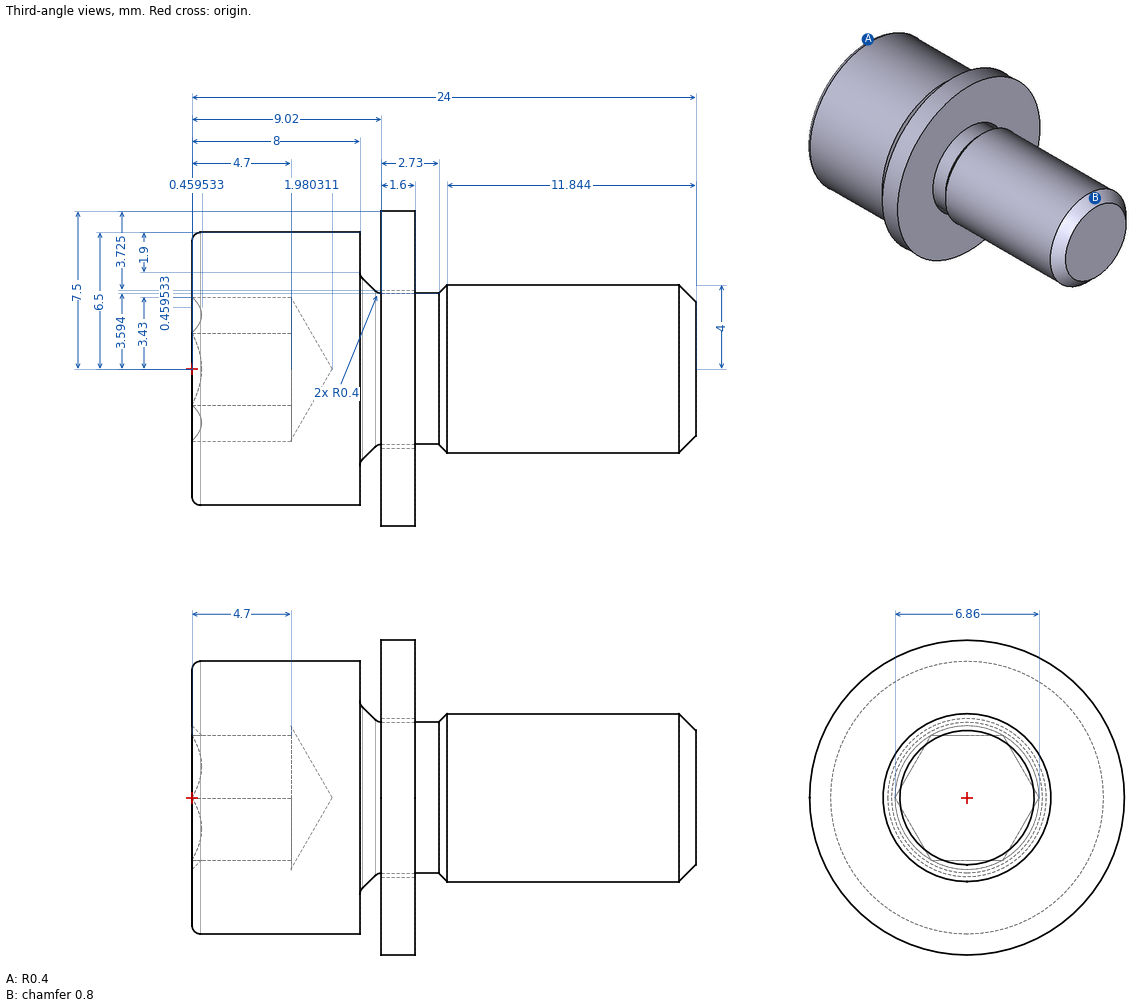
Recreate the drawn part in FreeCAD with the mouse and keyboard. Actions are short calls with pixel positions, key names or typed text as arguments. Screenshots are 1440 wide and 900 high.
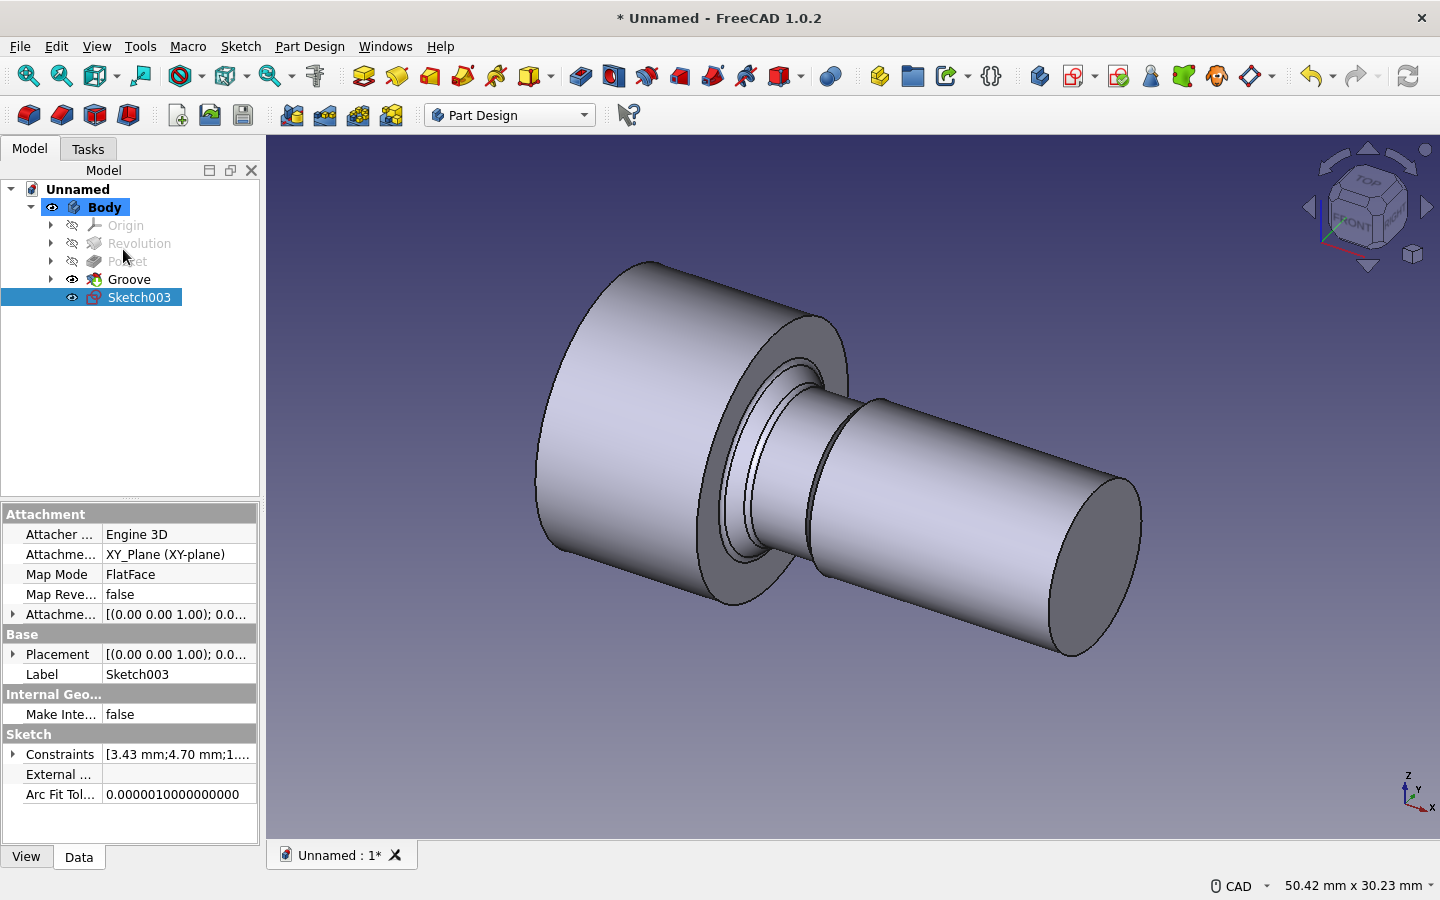
click(647, 76)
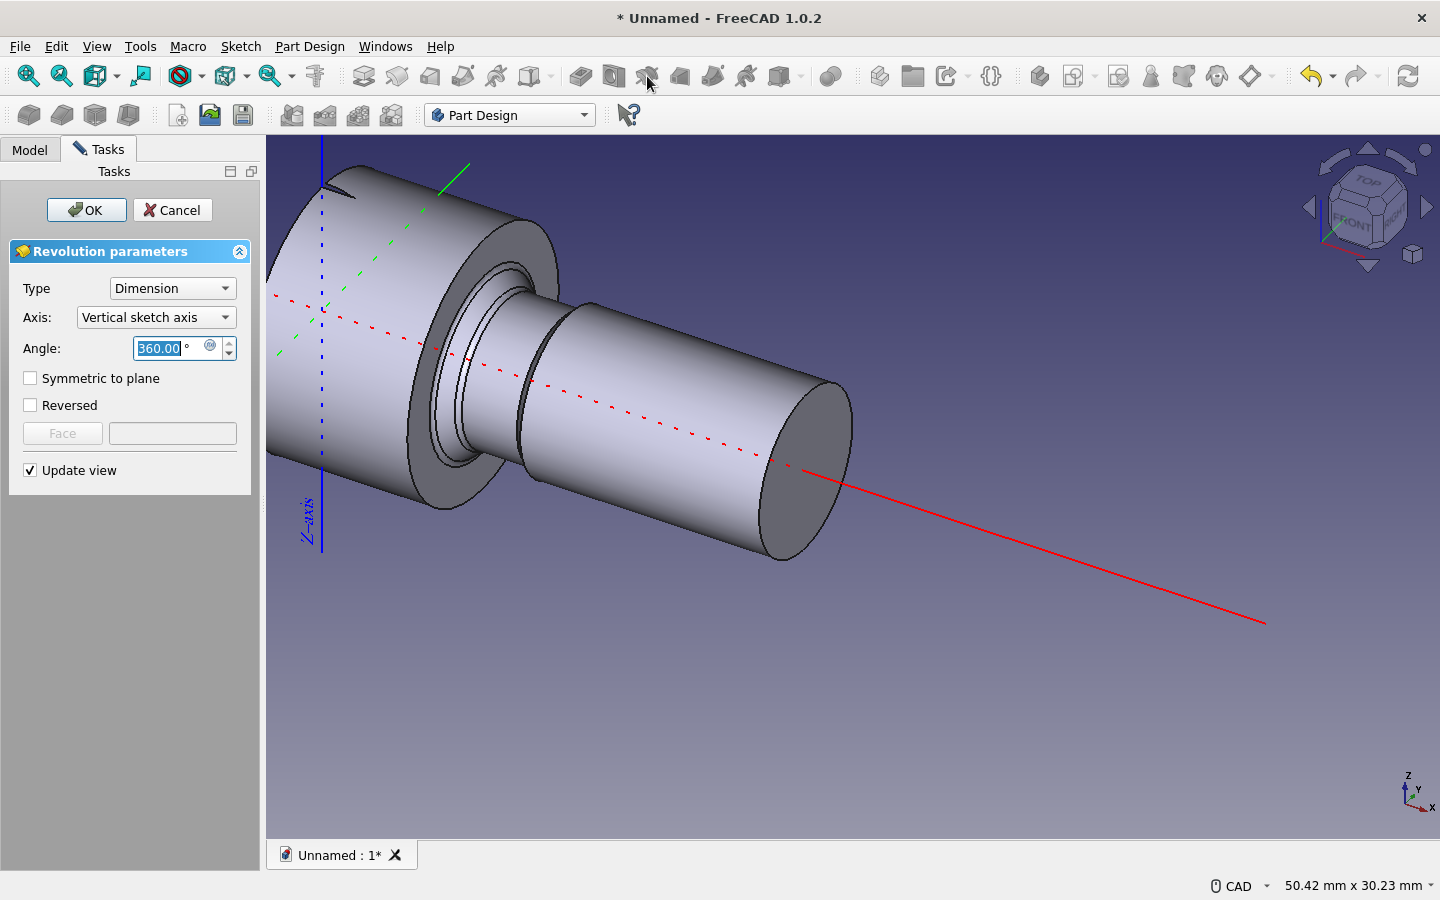
click(157, 318)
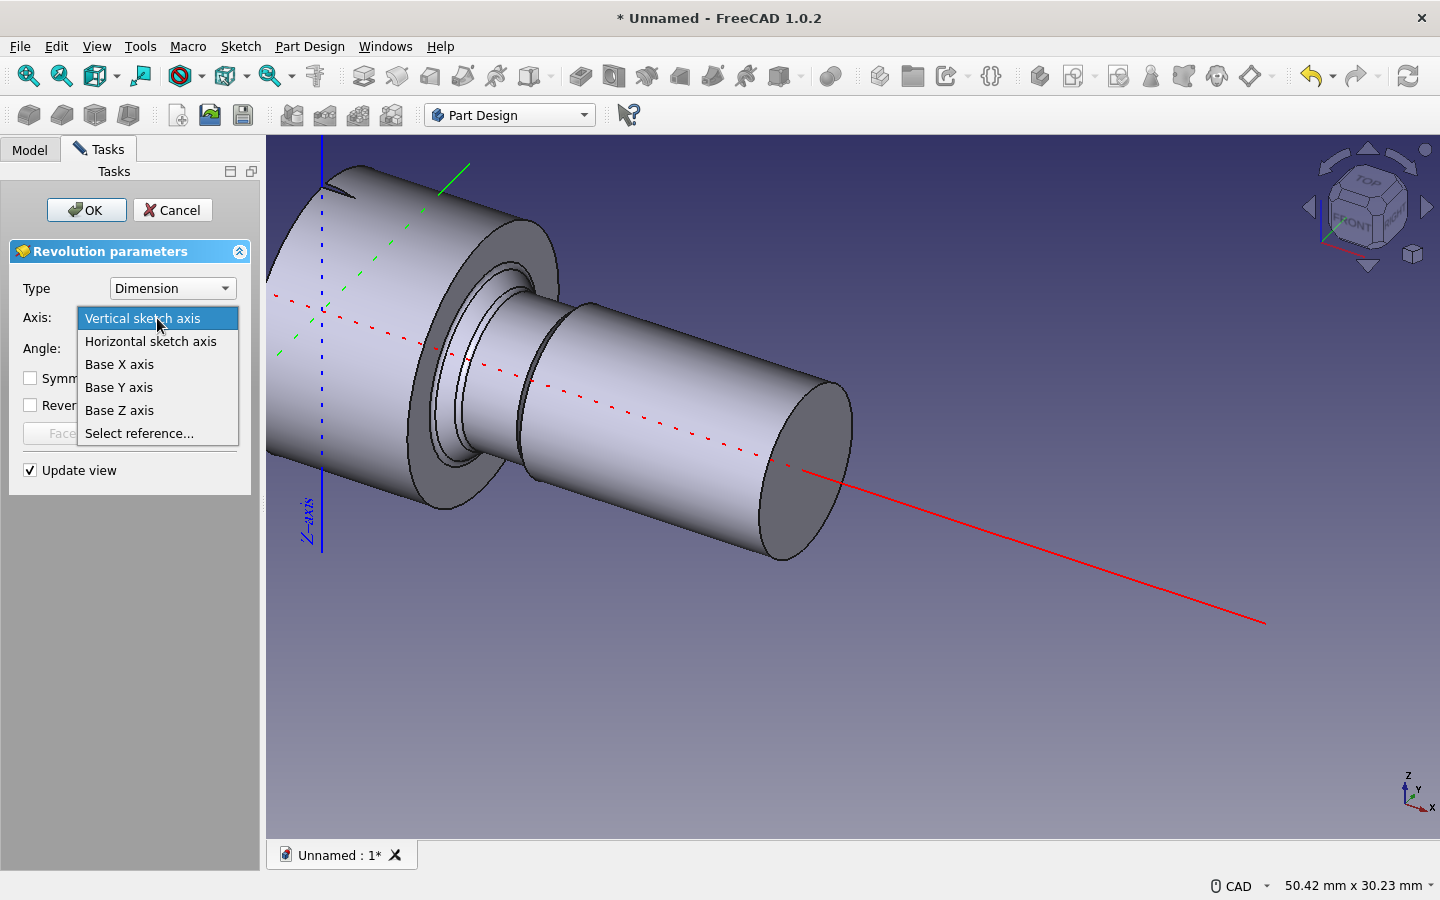
click(156, 342)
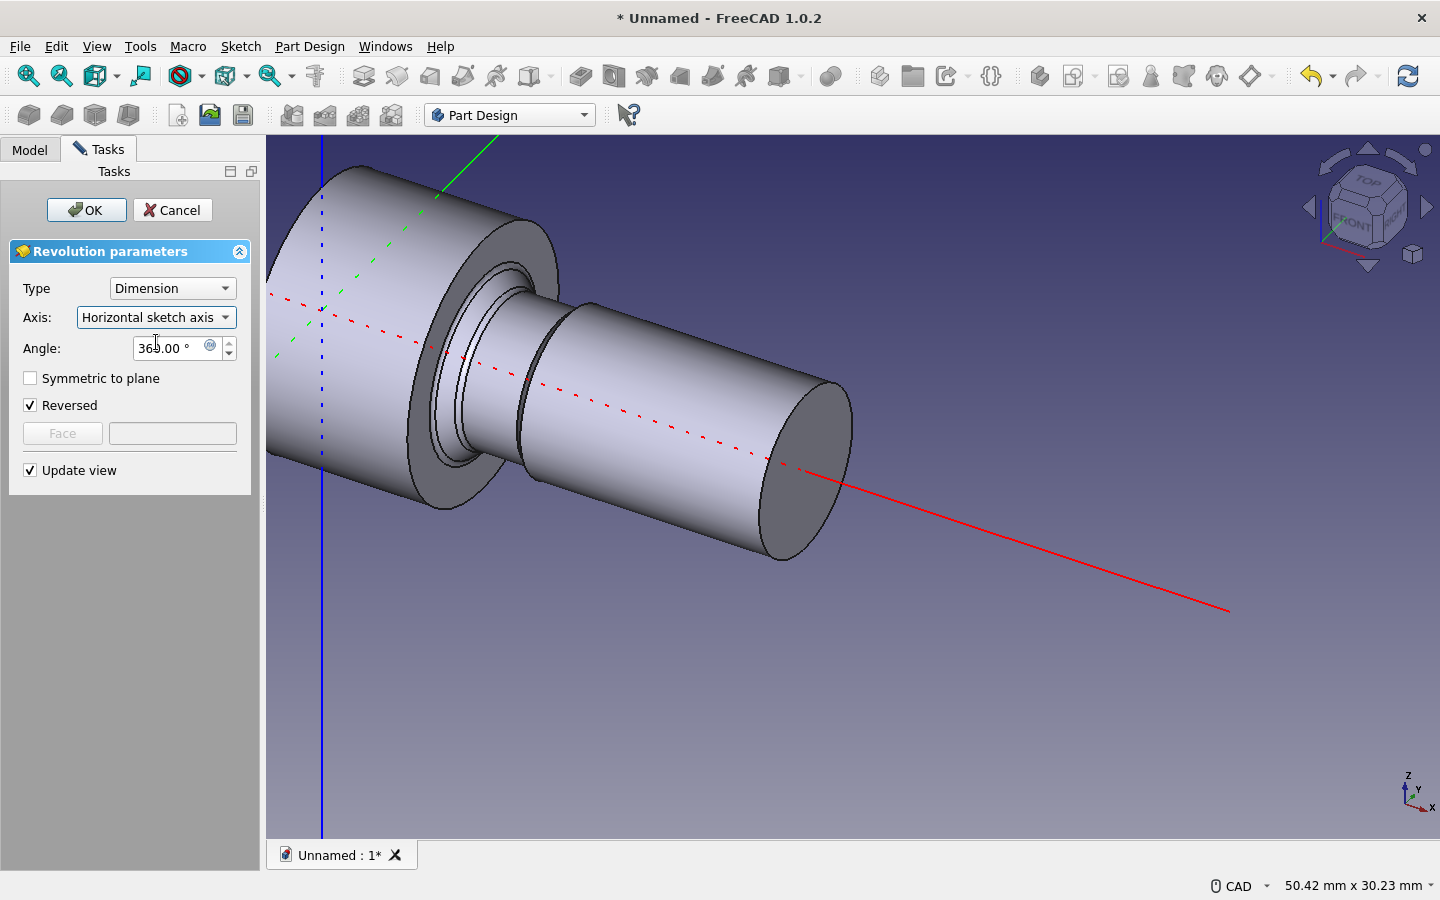
click(87, 210)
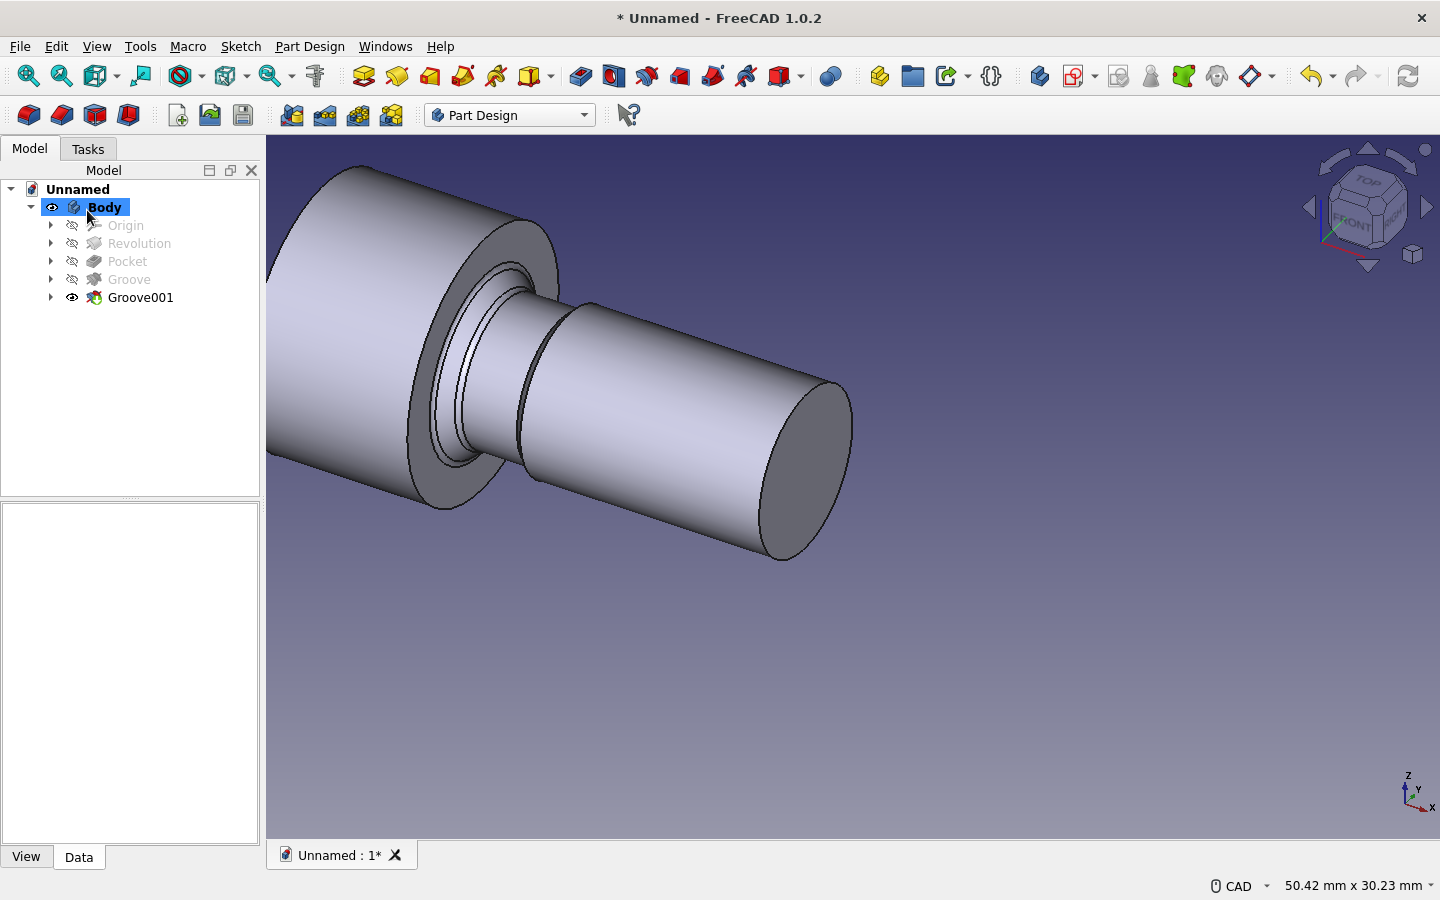
click(29, 76)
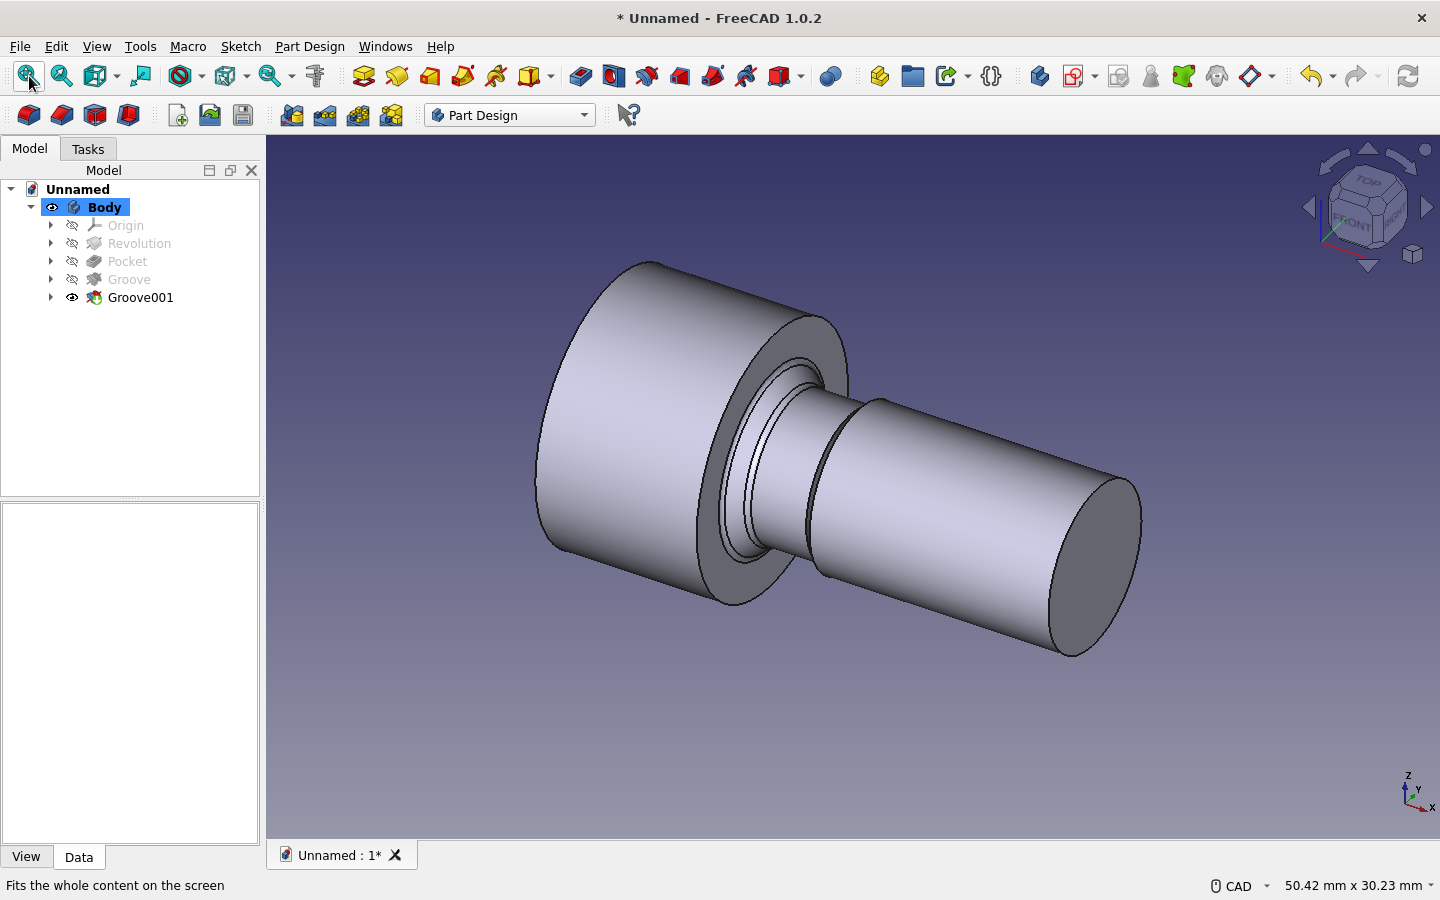
key(0)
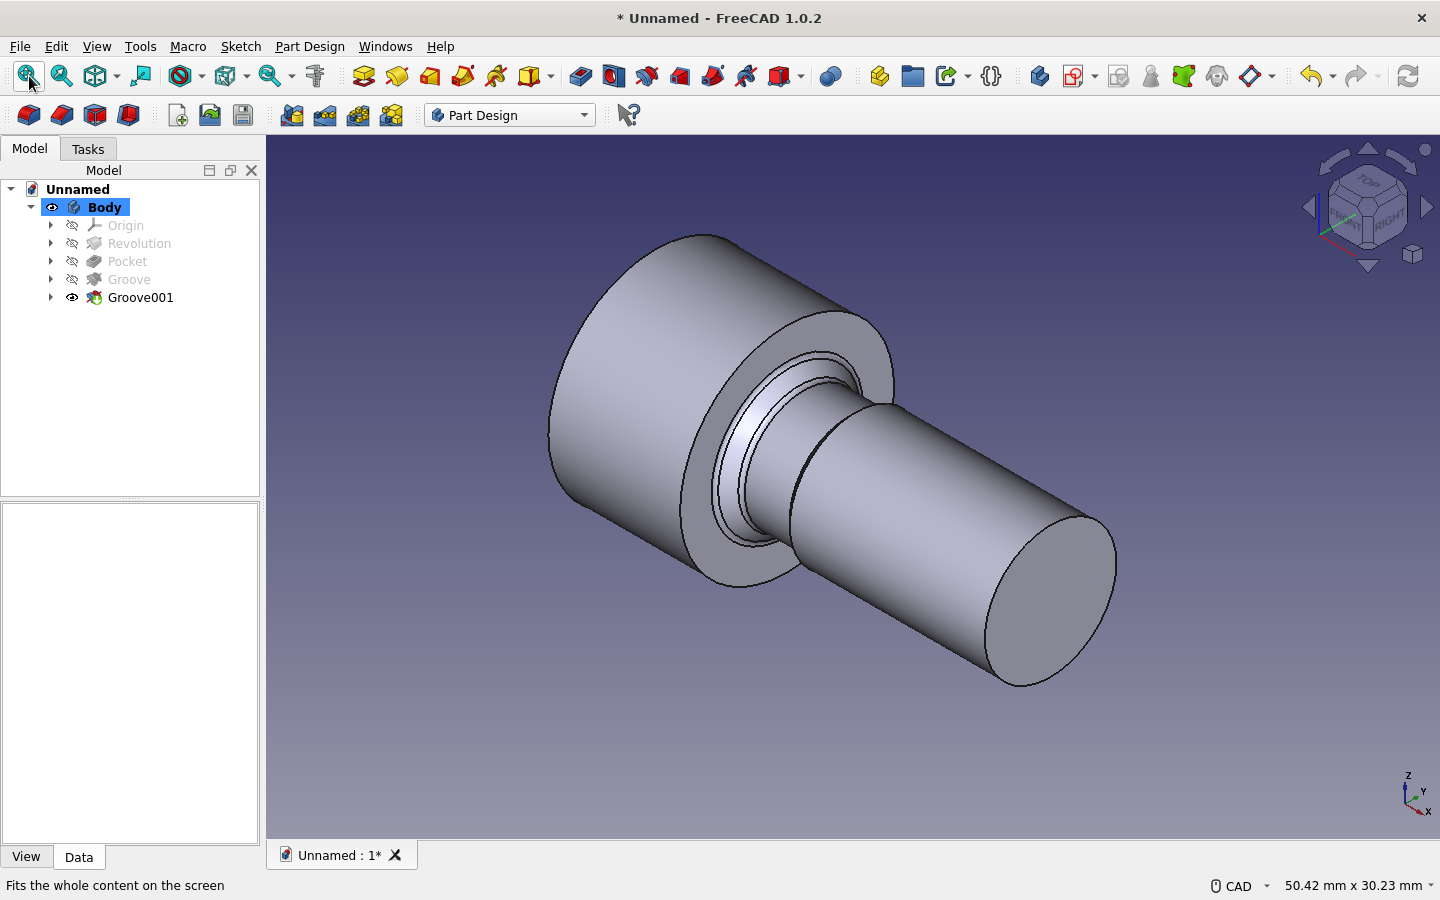
click(688, 235)